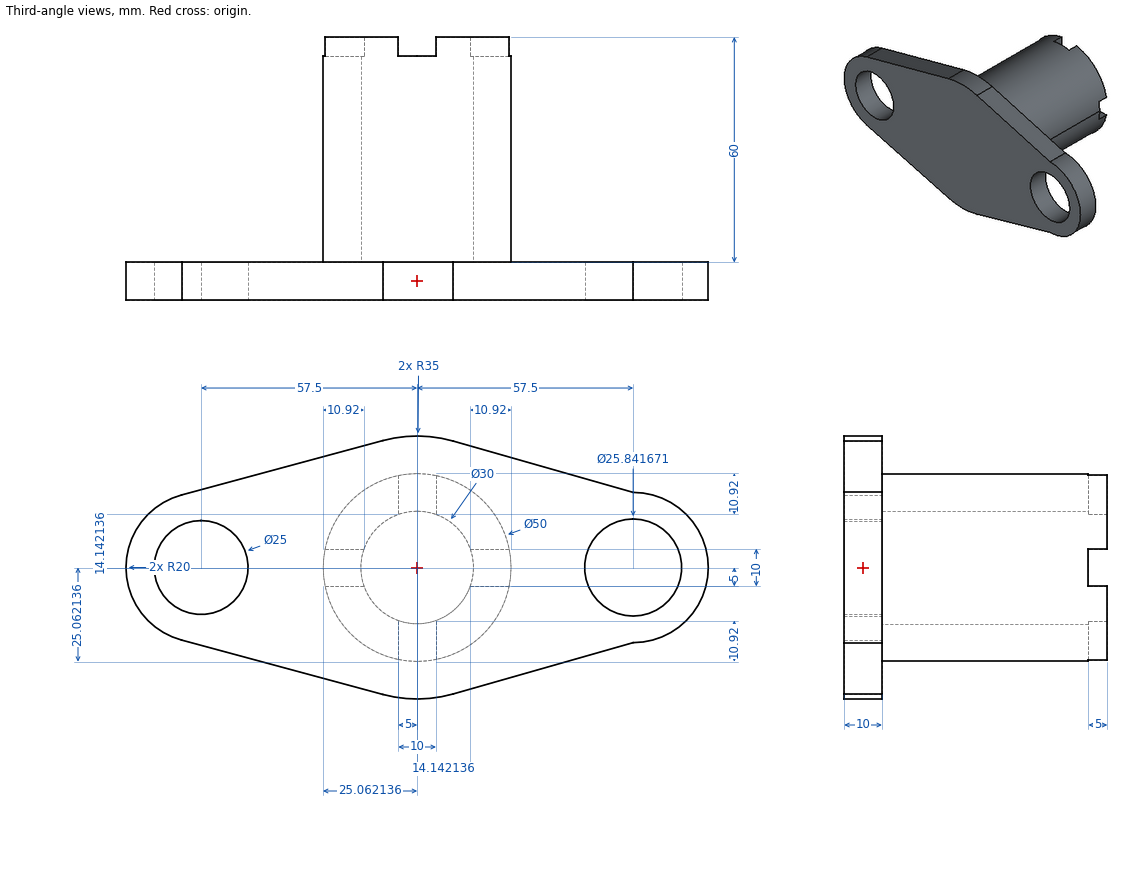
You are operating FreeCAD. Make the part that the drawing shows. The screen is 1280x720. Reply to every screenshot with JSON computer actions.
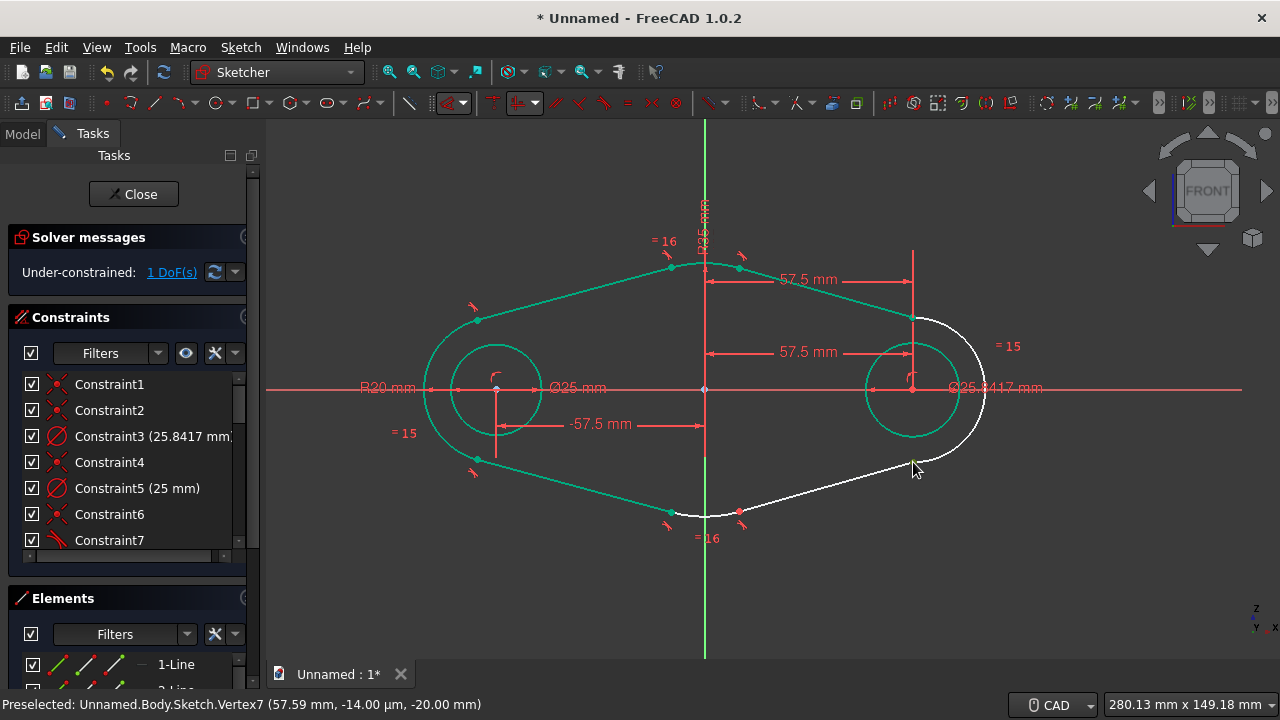
{"action": "key", "text": "l"}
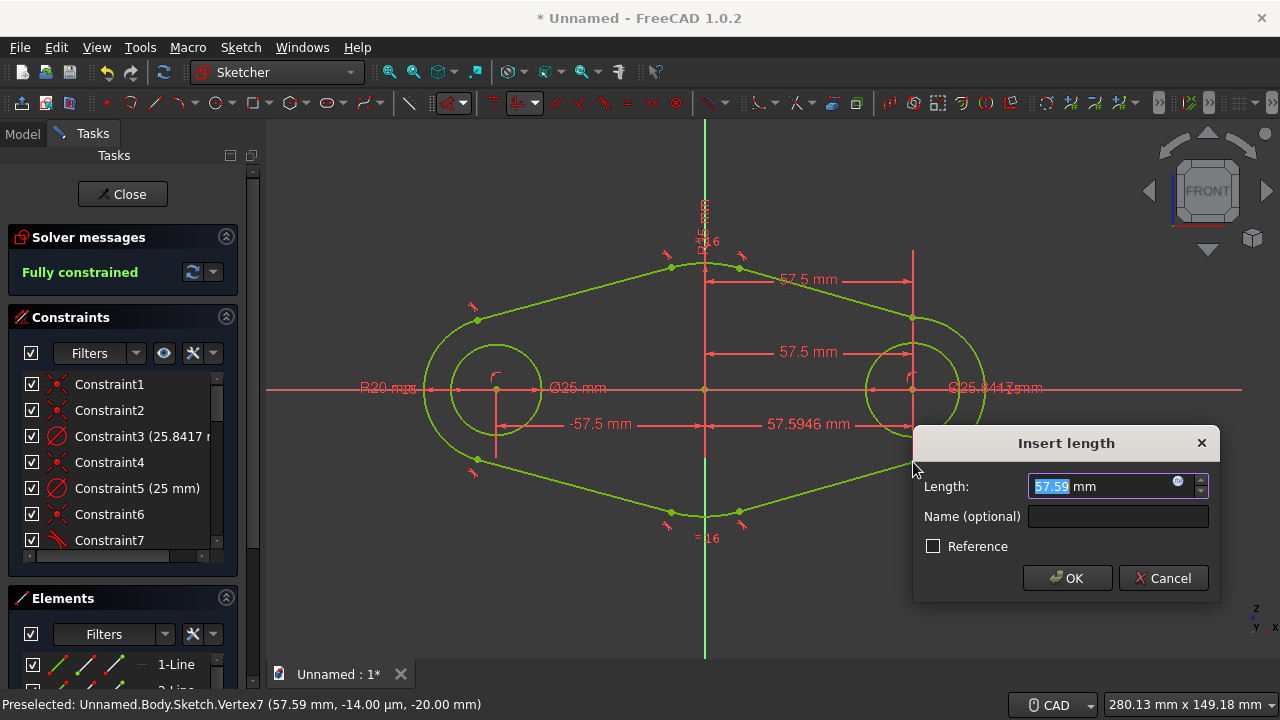
{"action": "type", "text": "57.5"}
{"action": "key", "text": "Return"}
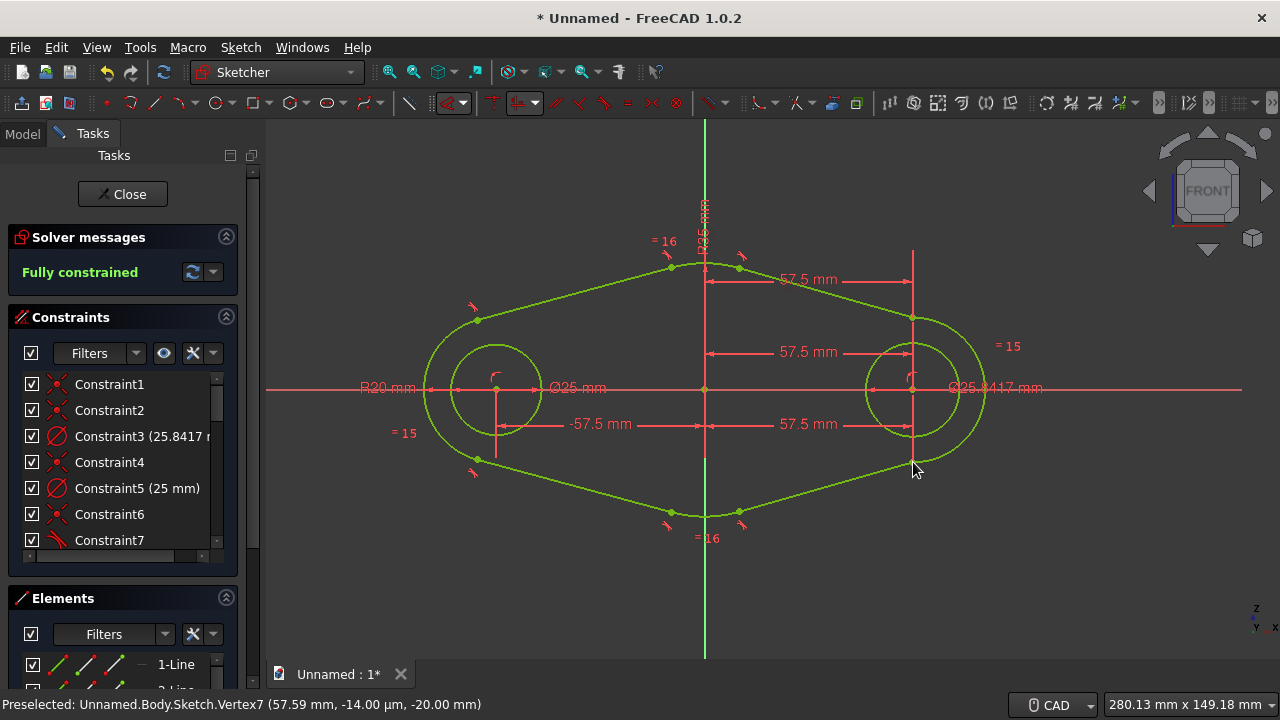
{"action": "left_click", "coordinate": [123, 194]}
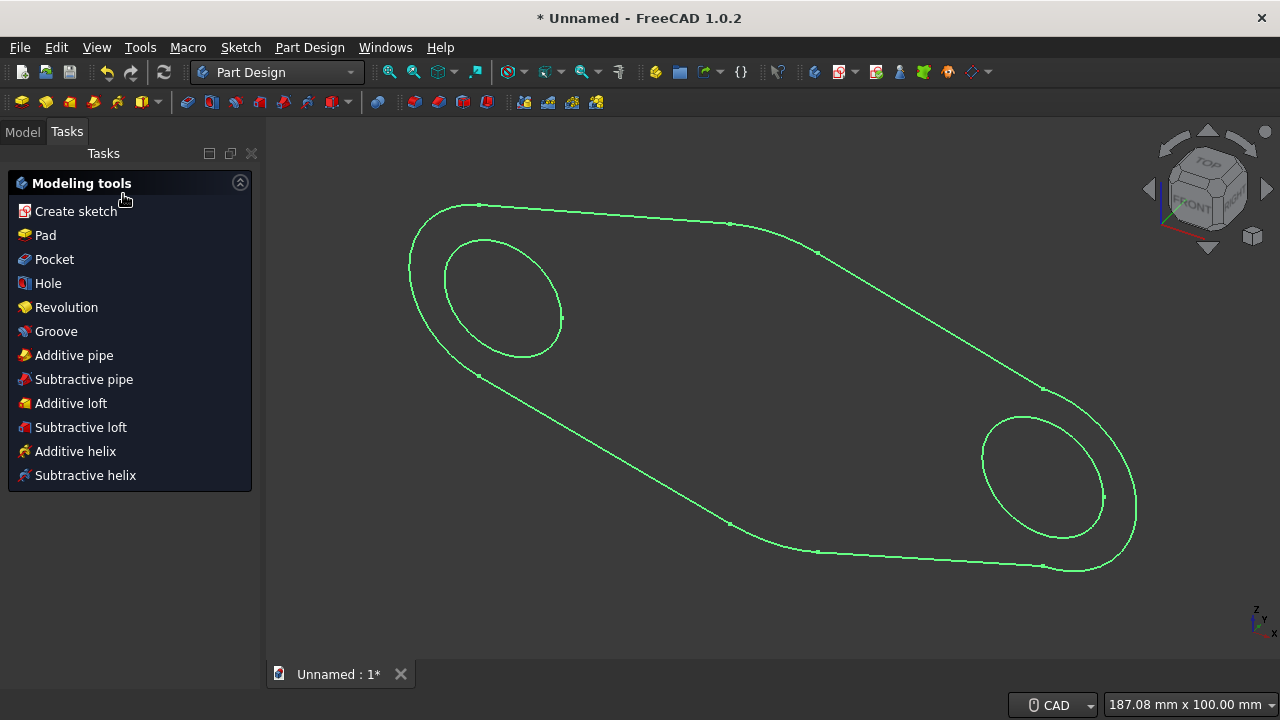
{"action": "left_click", "coordinate": [22, 102]}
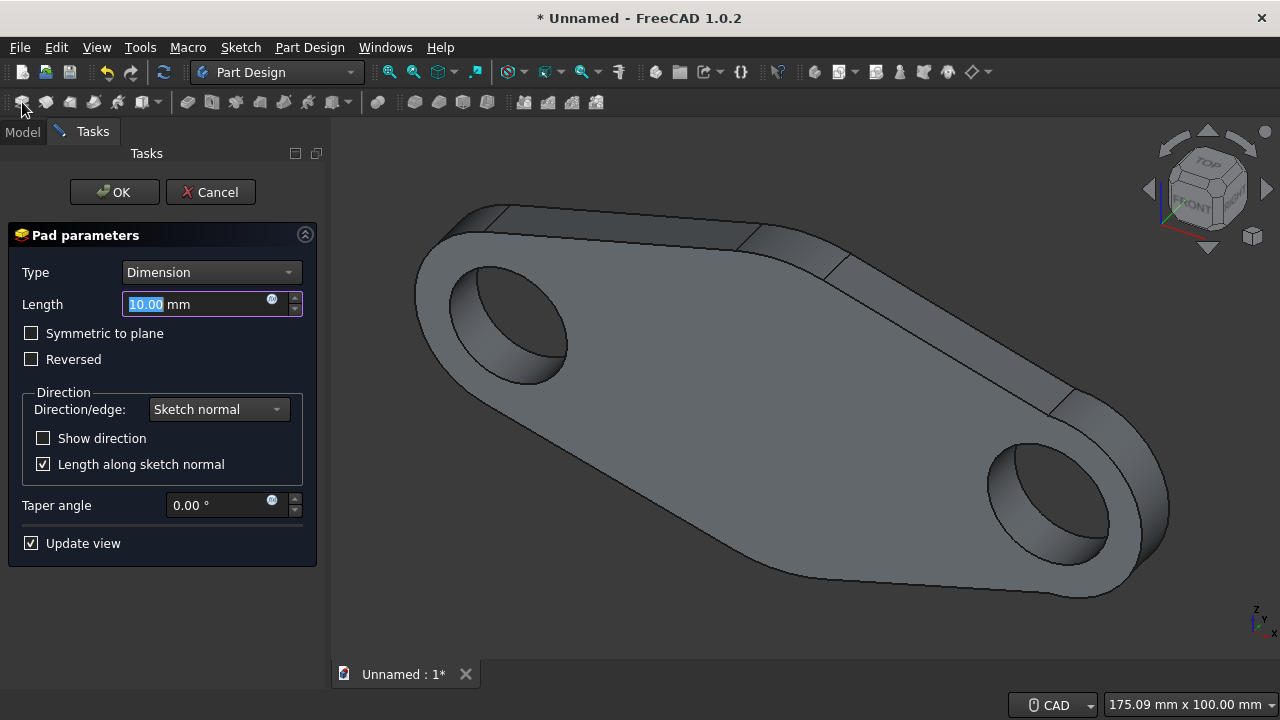
{"action": "type", "text": "10"}
{"action": "key", "text": "Tab"}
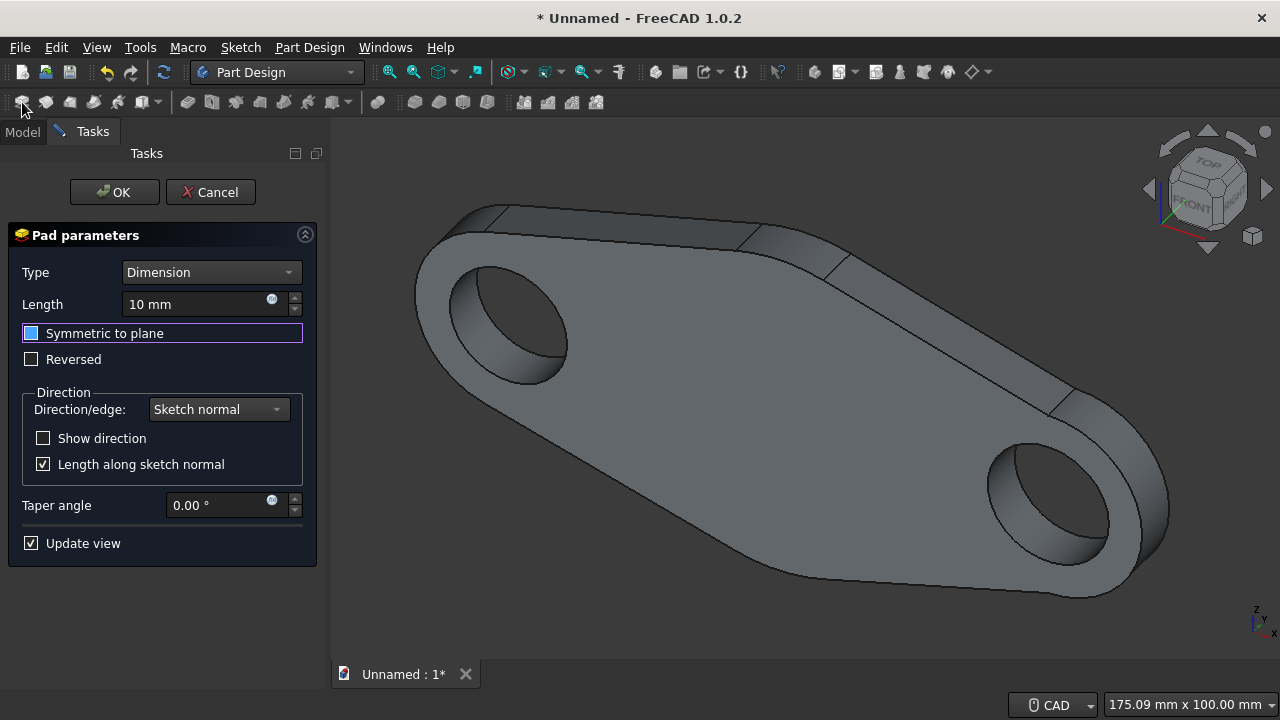
{"action": "left_click", "coordinate": [30, 333]}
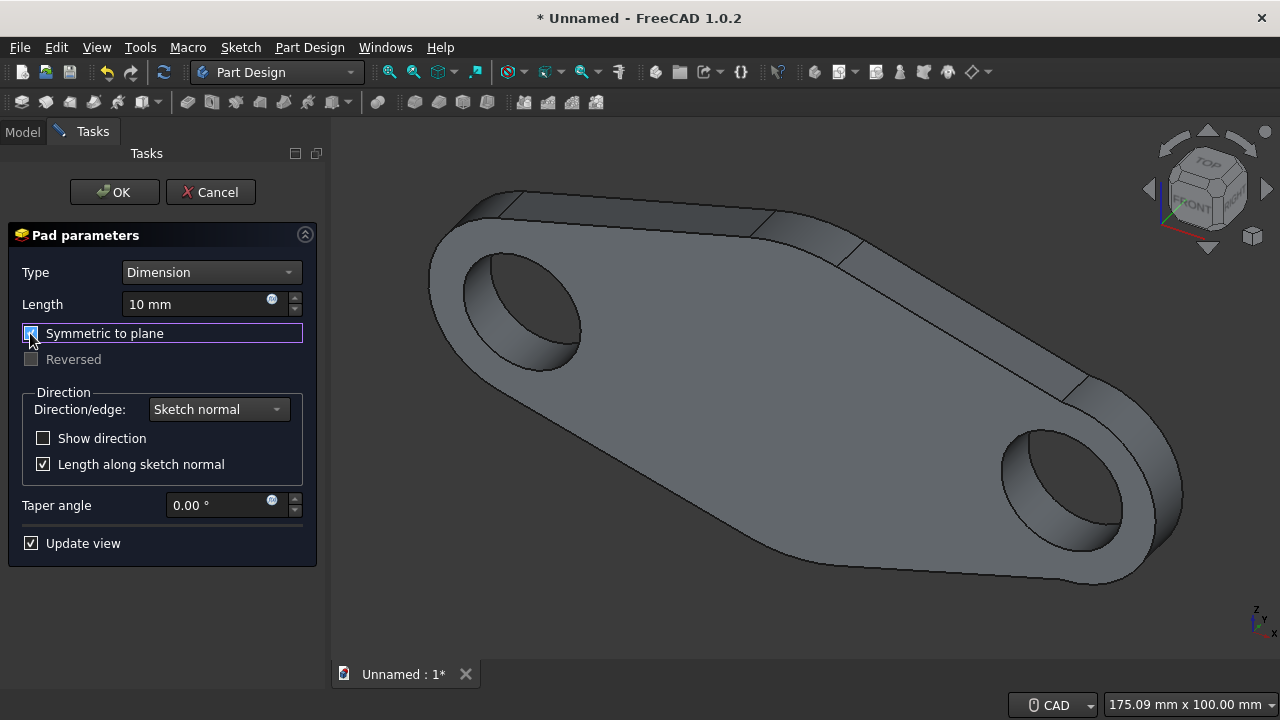
{"action": "left_click", "coordinate": [115, 192]}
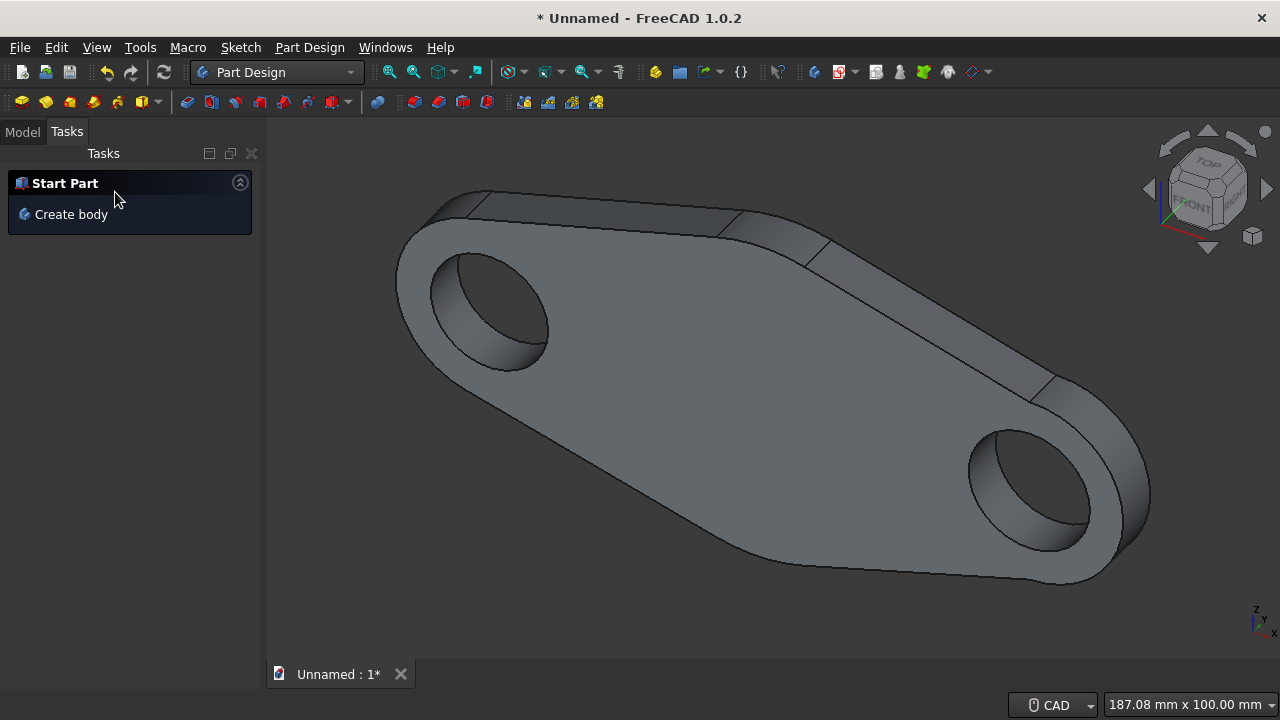
{"action": "left_click", "coordinate": [390, 72]}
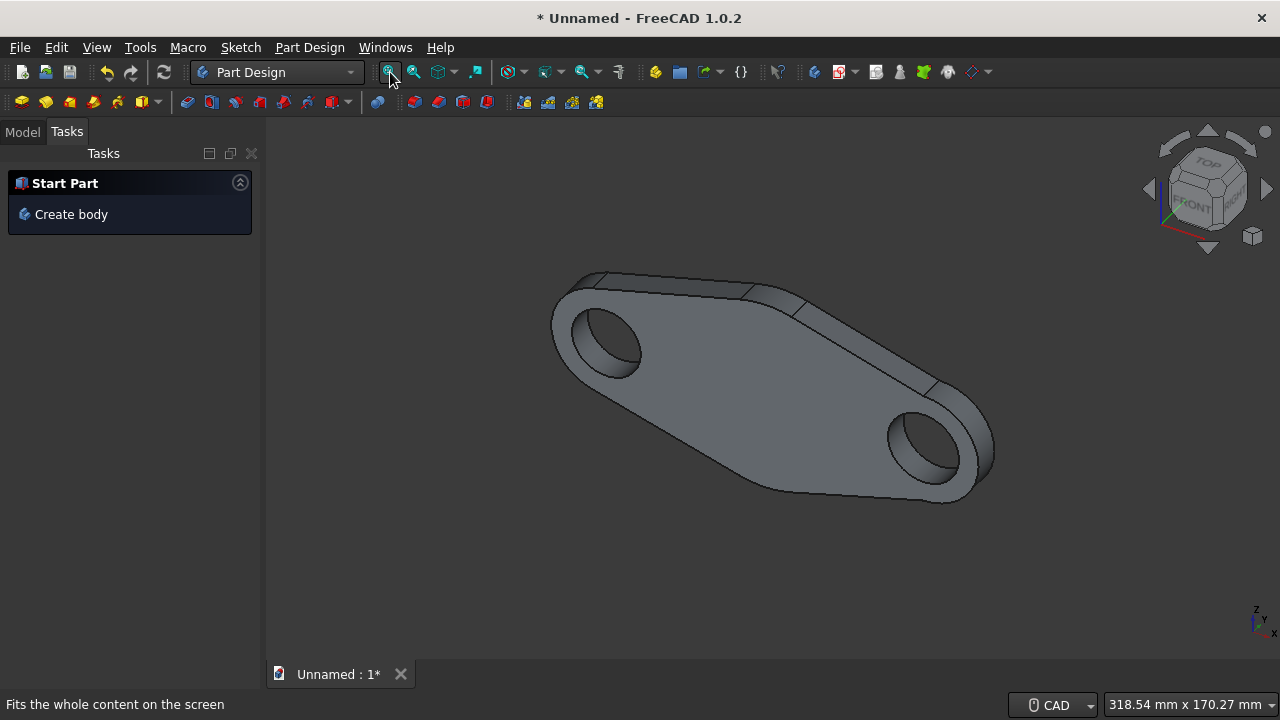
{"action": "key", "text": "4"}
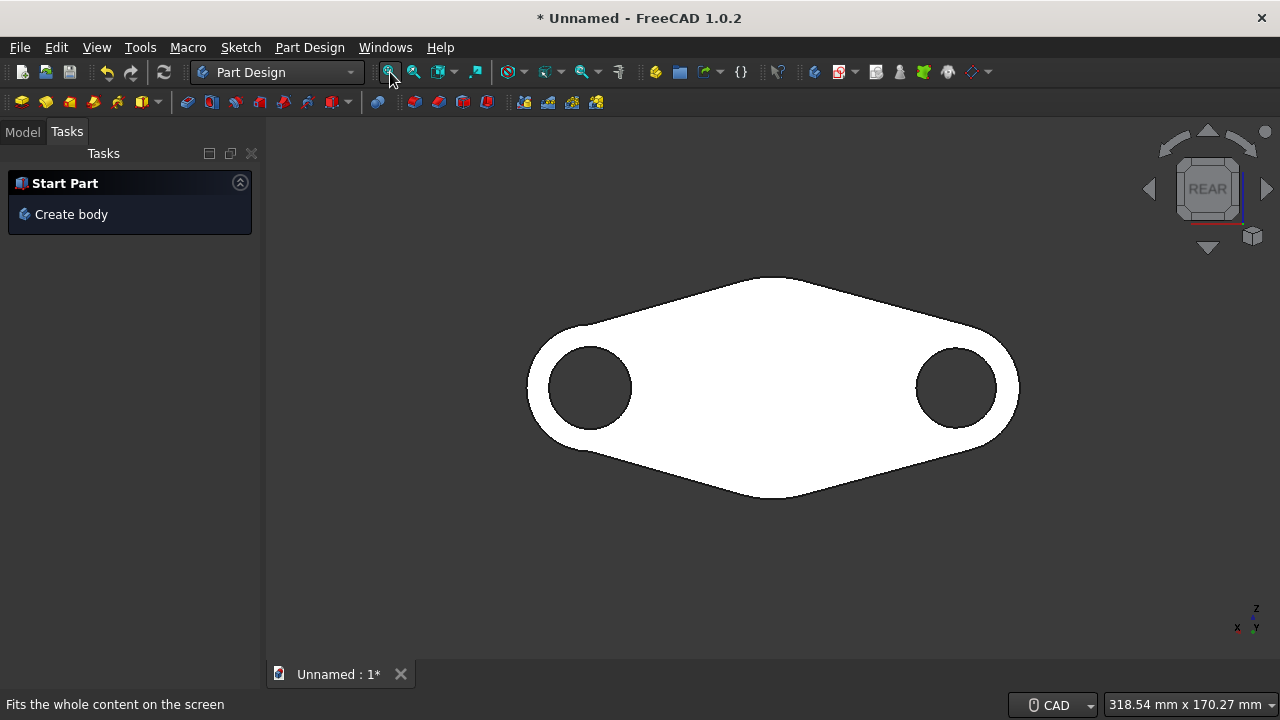
{"action": "left_click", "coordinate": [773, 387]}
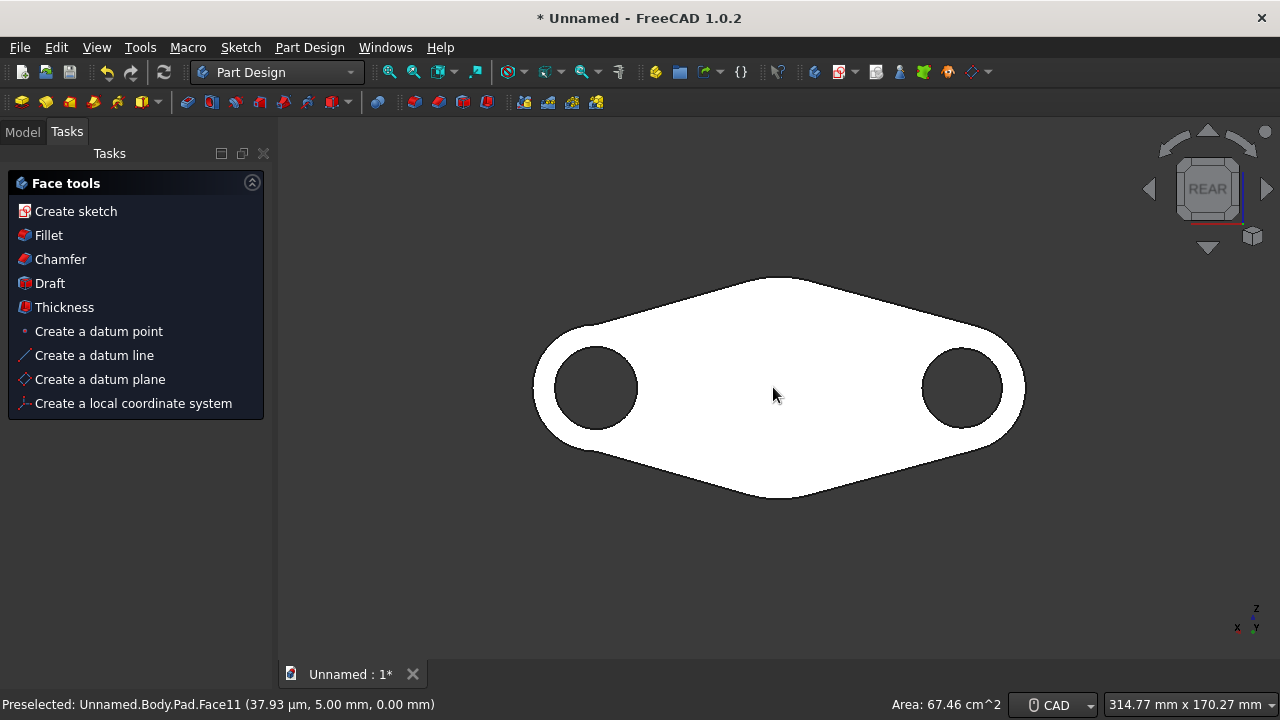
{"action": "left_click", "coordinate": [840, 72]}